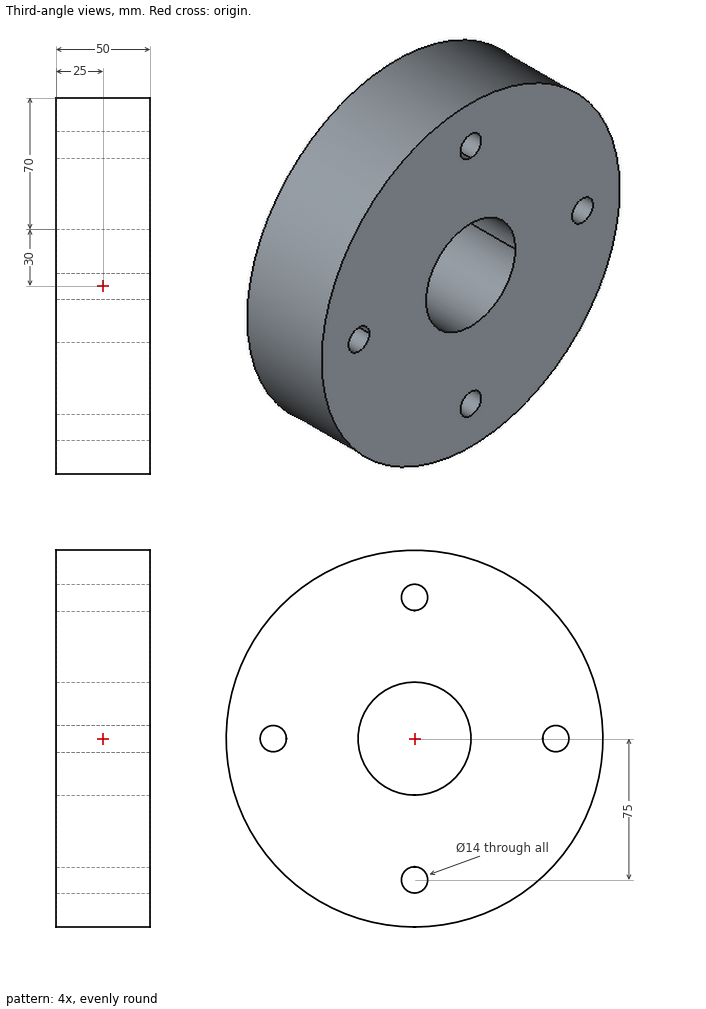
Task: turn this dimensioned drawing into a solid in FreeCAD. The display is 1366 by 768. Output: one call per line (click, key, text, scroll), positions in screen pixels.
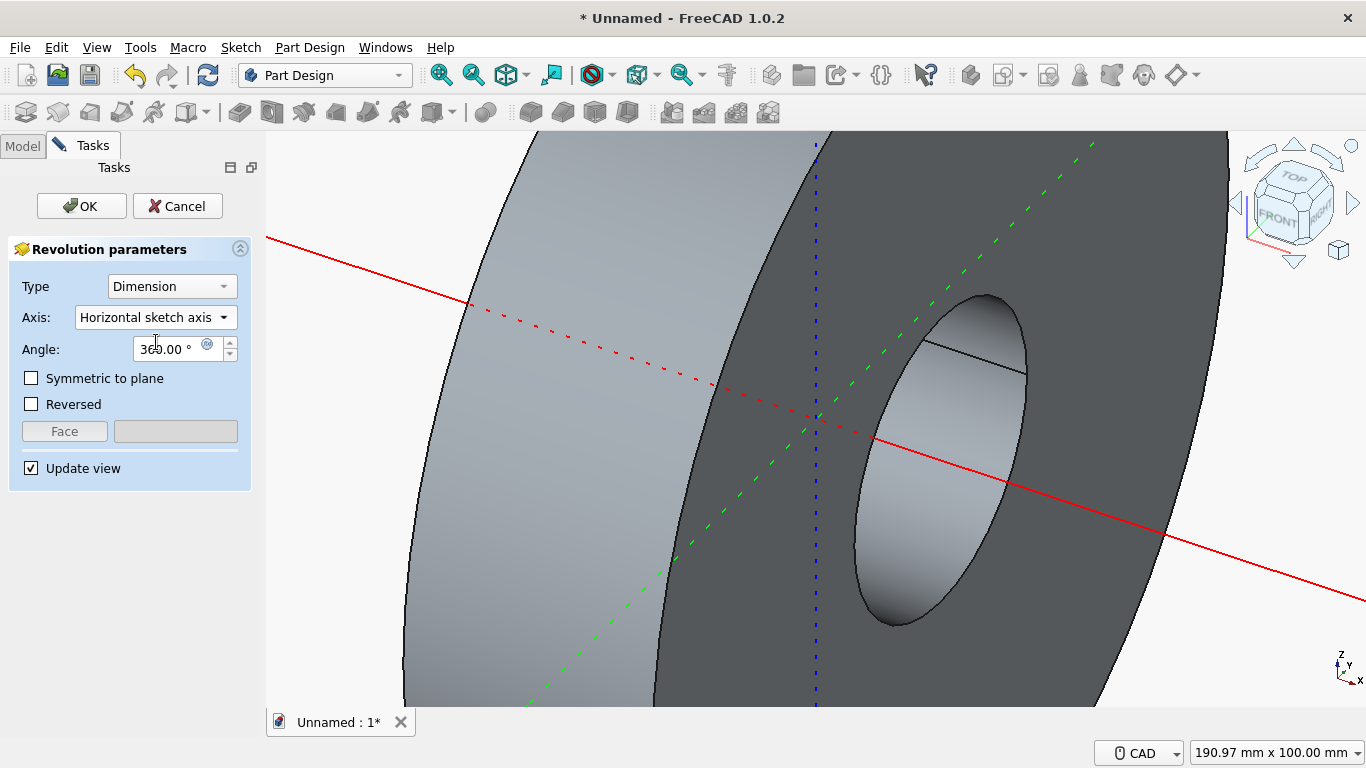
click(82, 206)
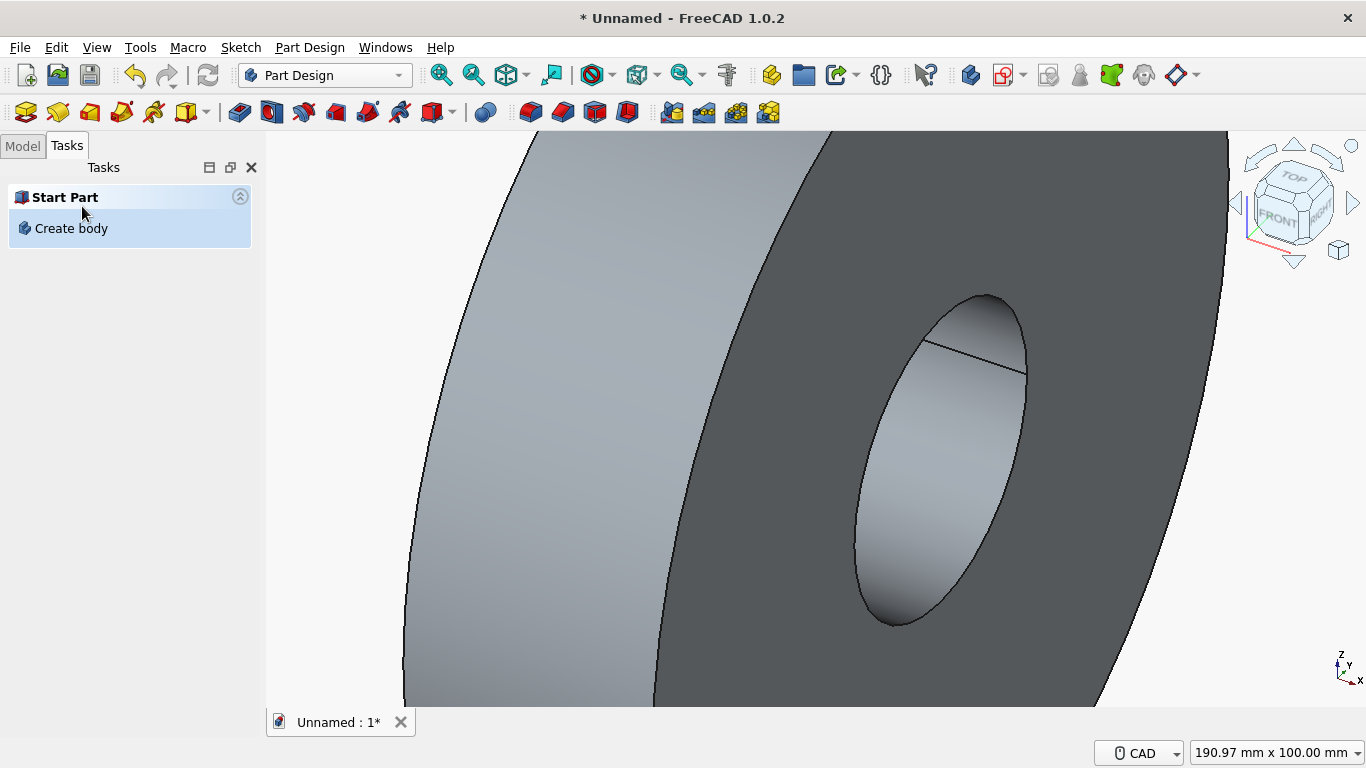
click(442, 76)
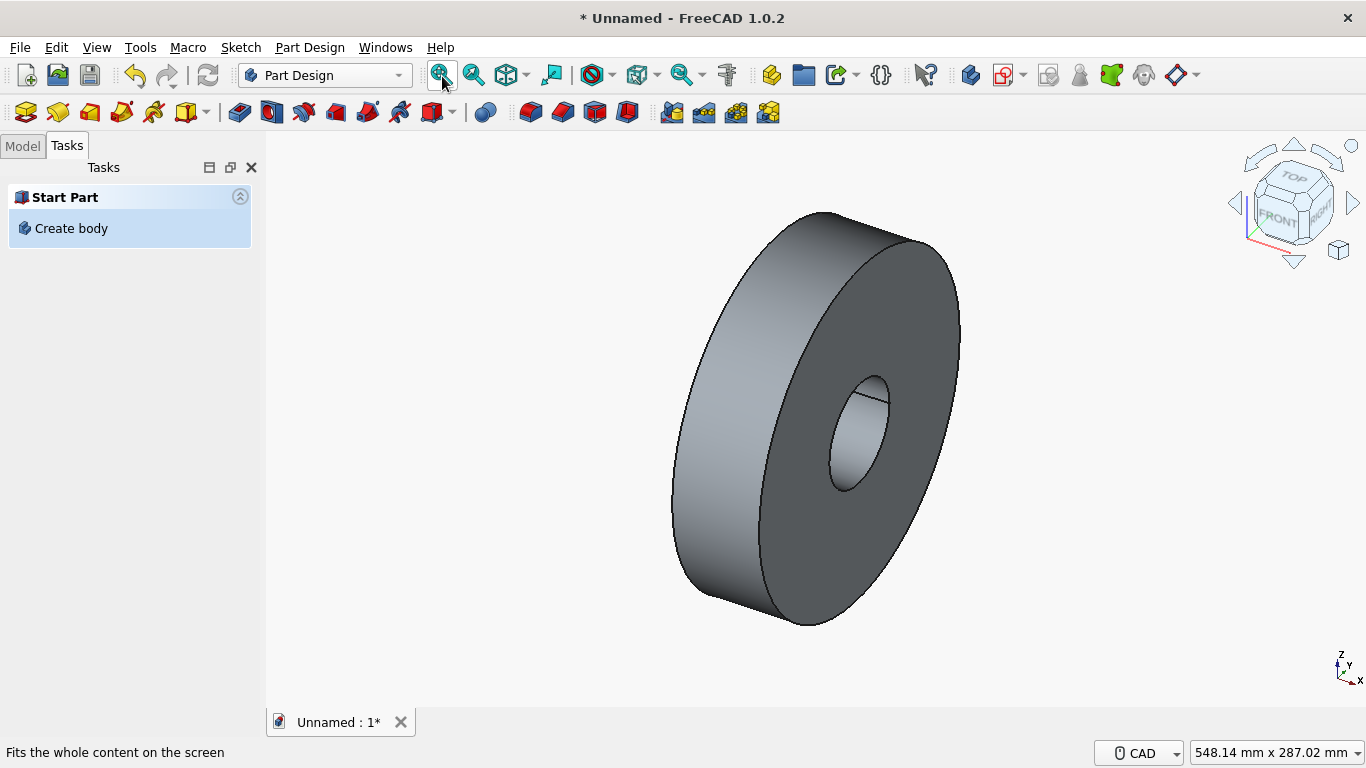
key(6)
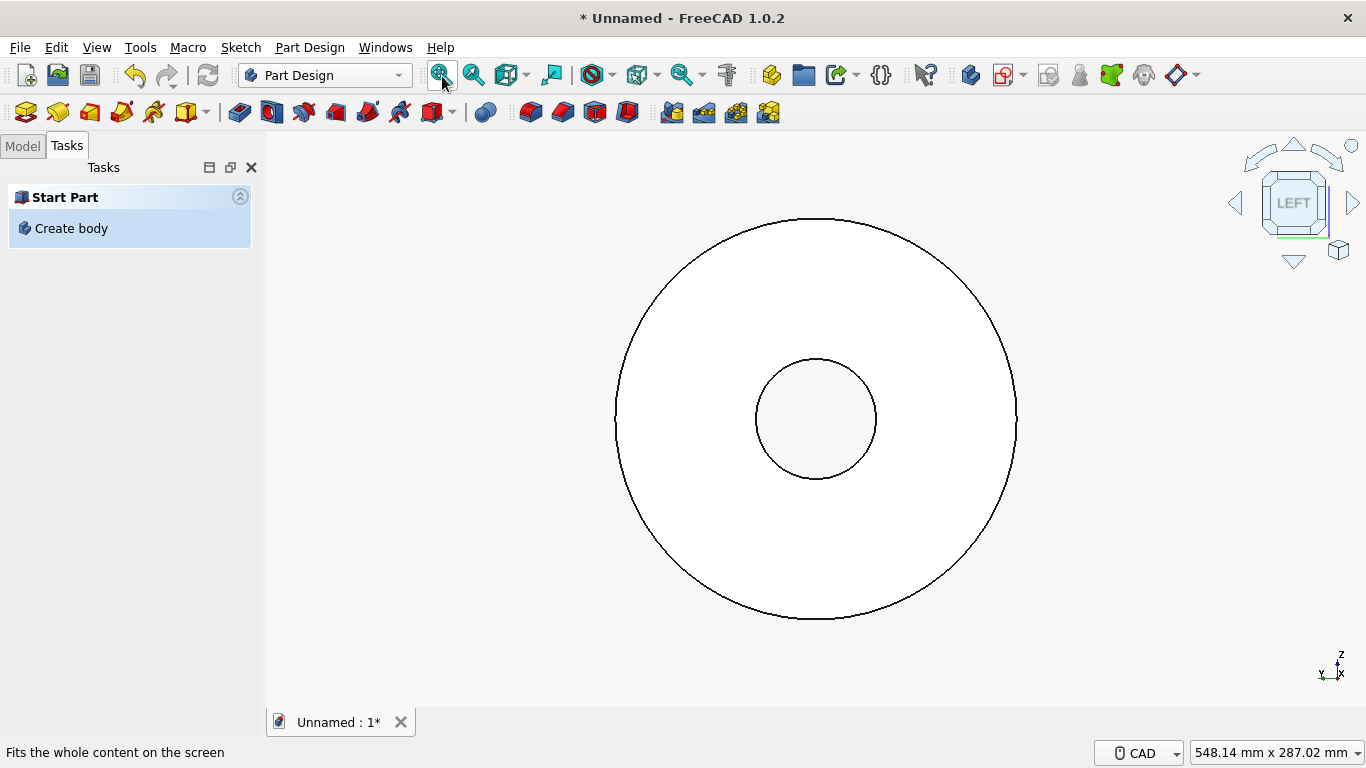
click(701, 361)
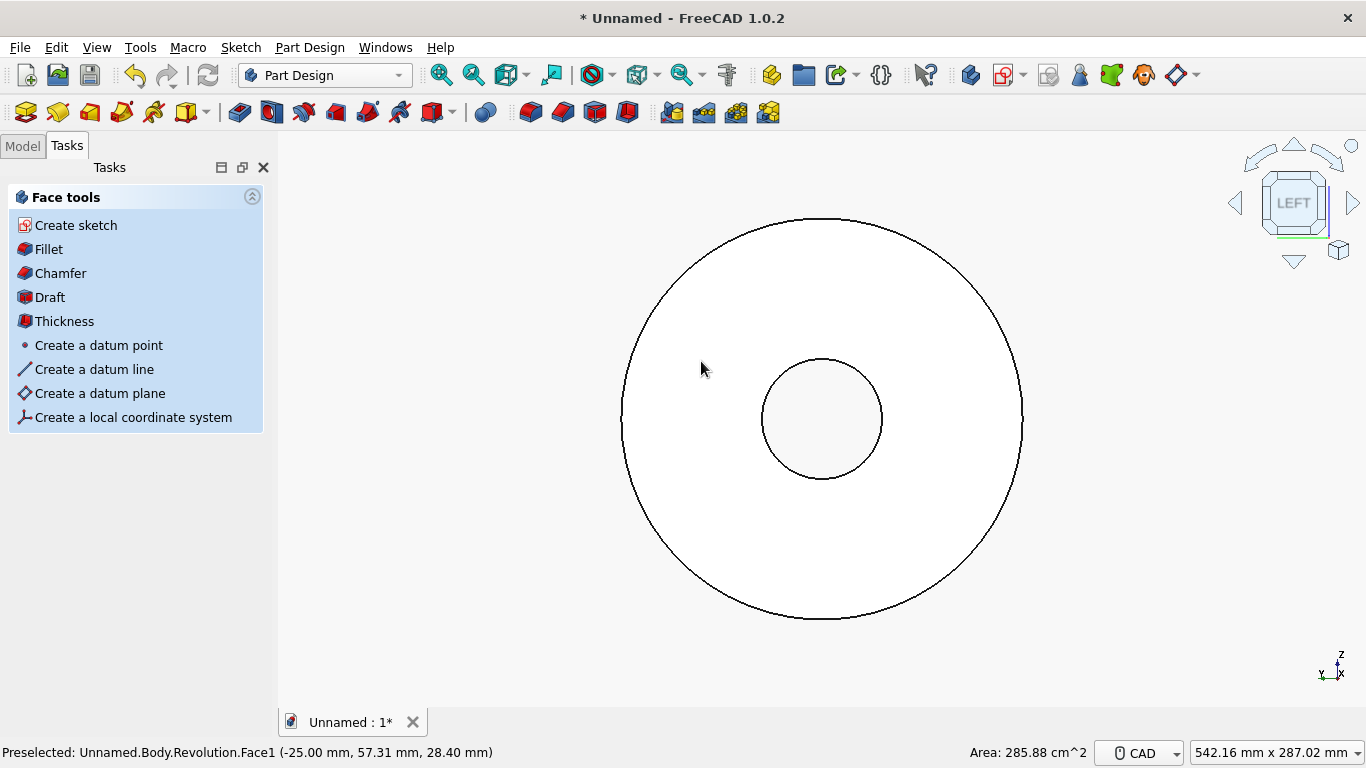
click(1004, 76)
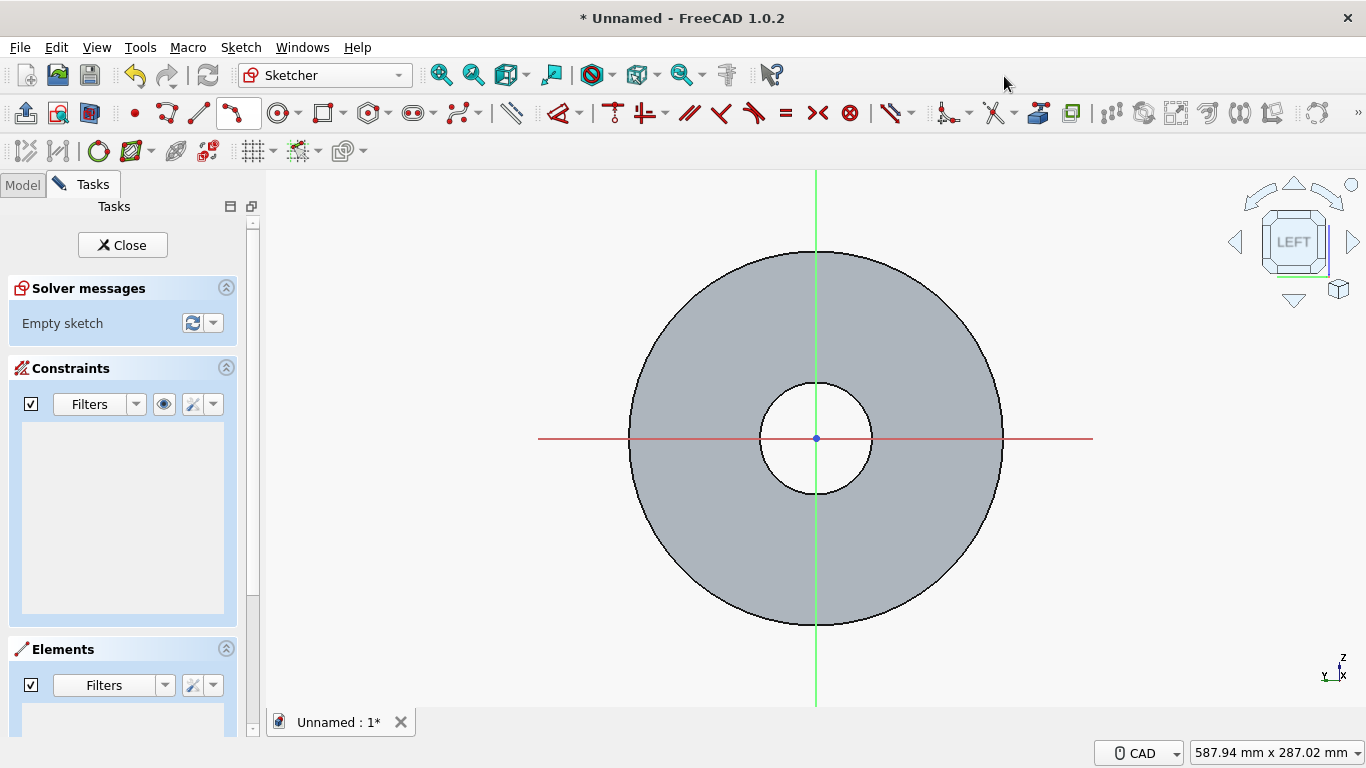
scroll(821, 590, up, 13)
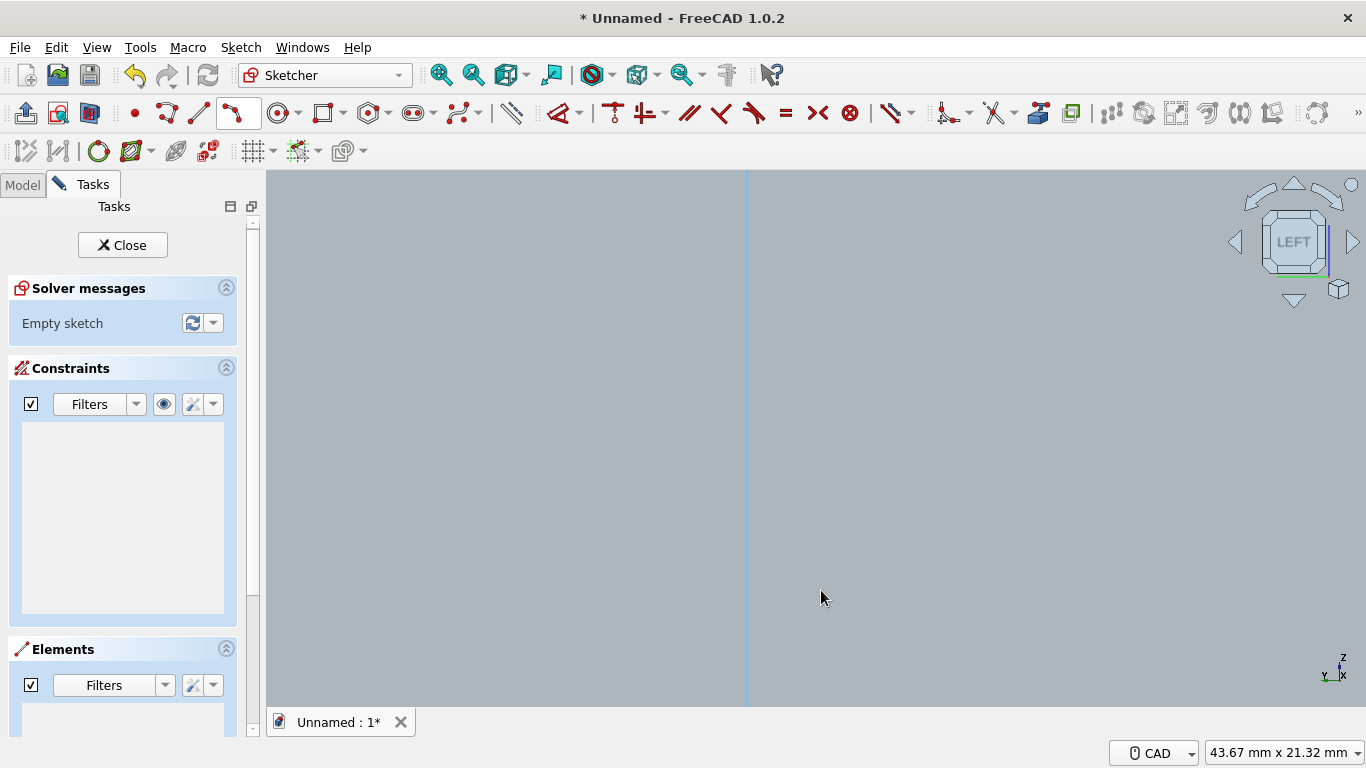
click(278, 114)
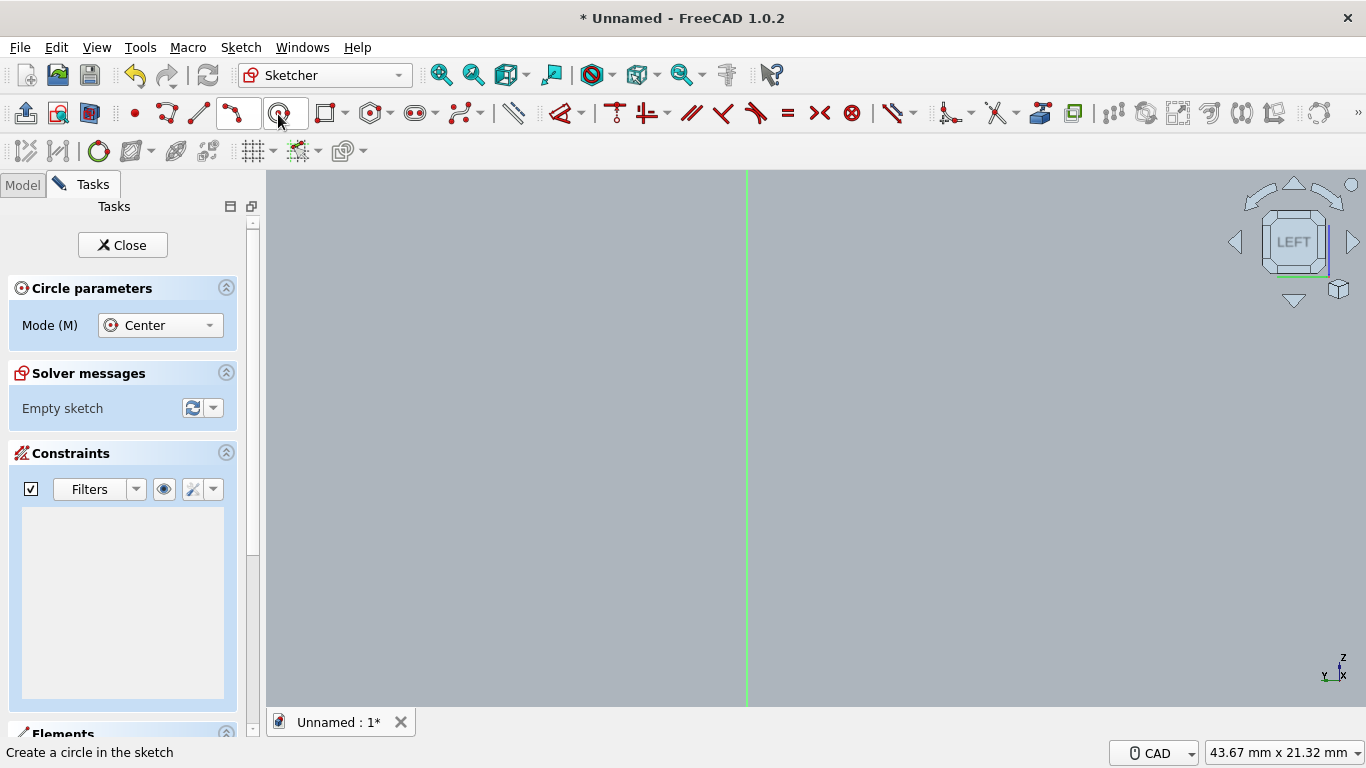
click(747, 430)
click(872, 305)
key(Escape)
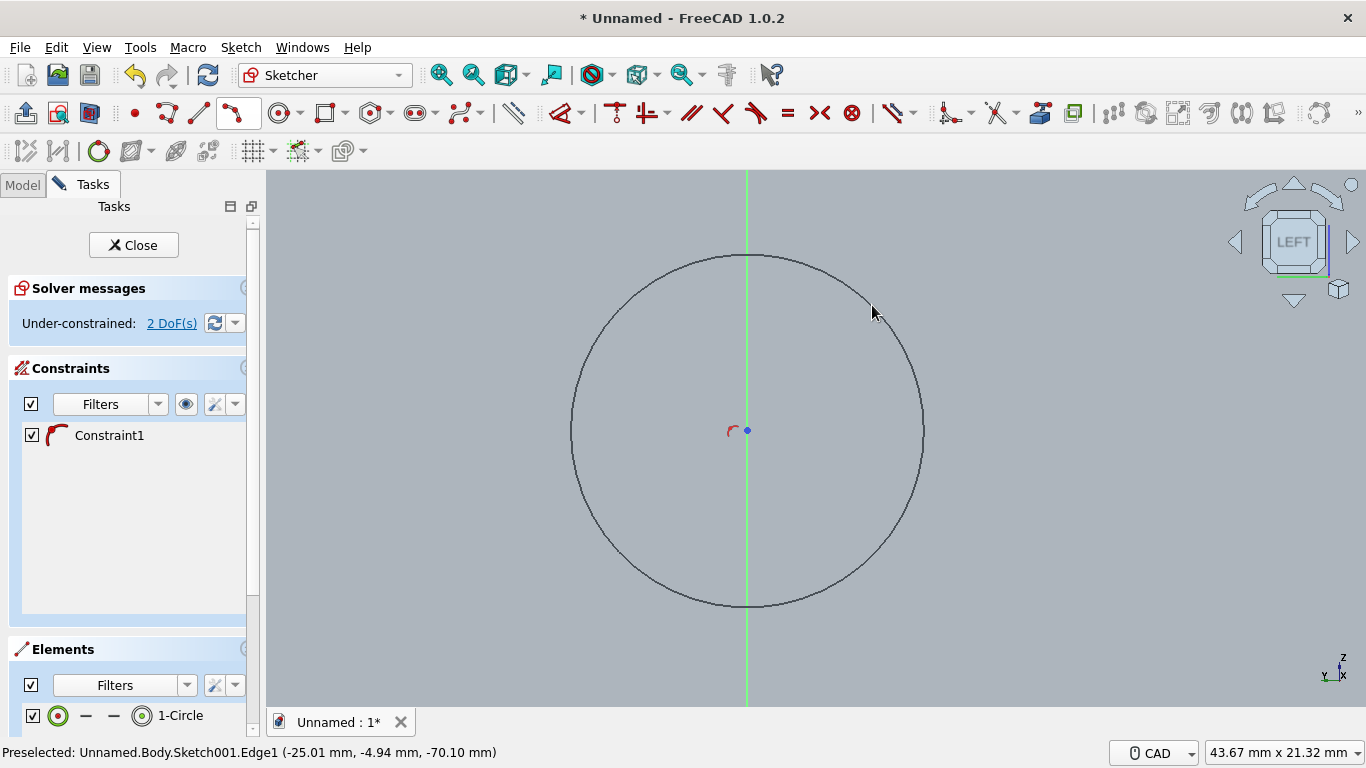
click(560, 114)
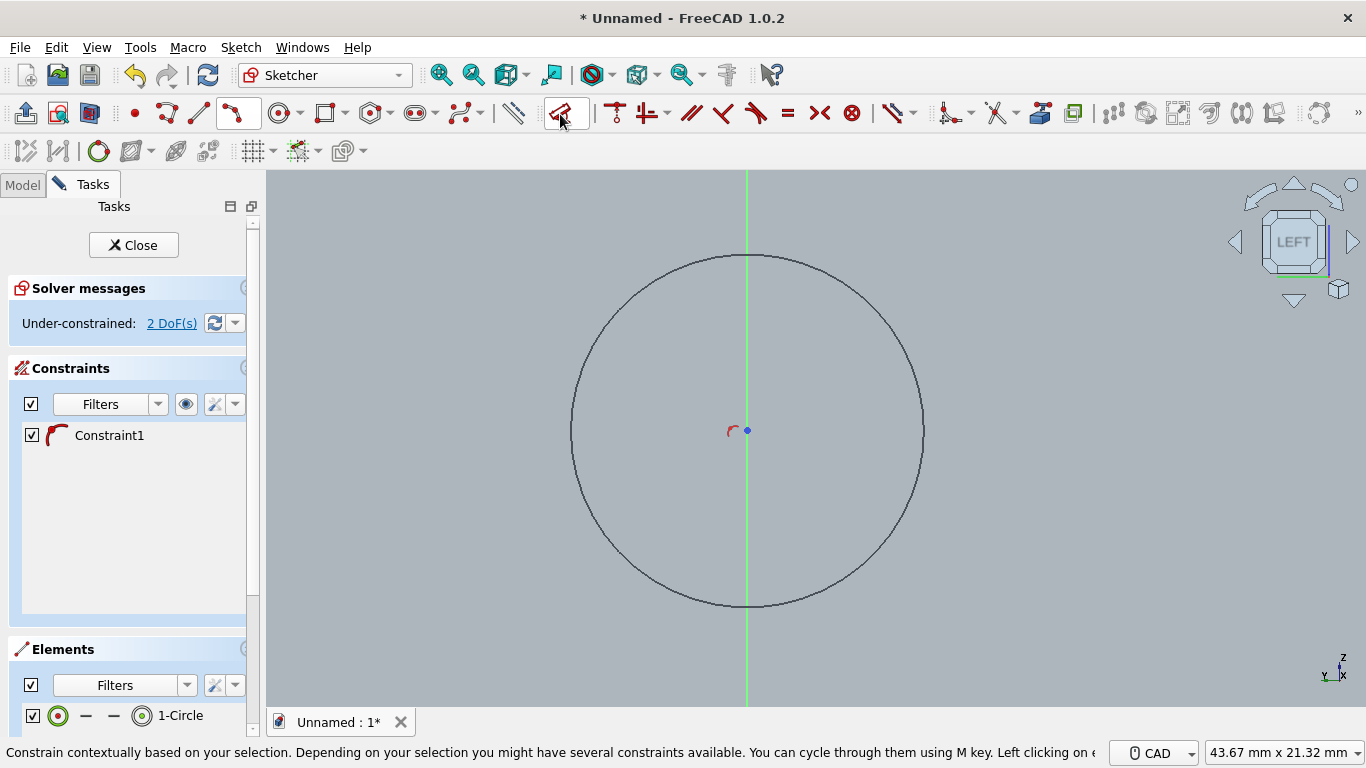
click(872, 306)
click(895, 283)